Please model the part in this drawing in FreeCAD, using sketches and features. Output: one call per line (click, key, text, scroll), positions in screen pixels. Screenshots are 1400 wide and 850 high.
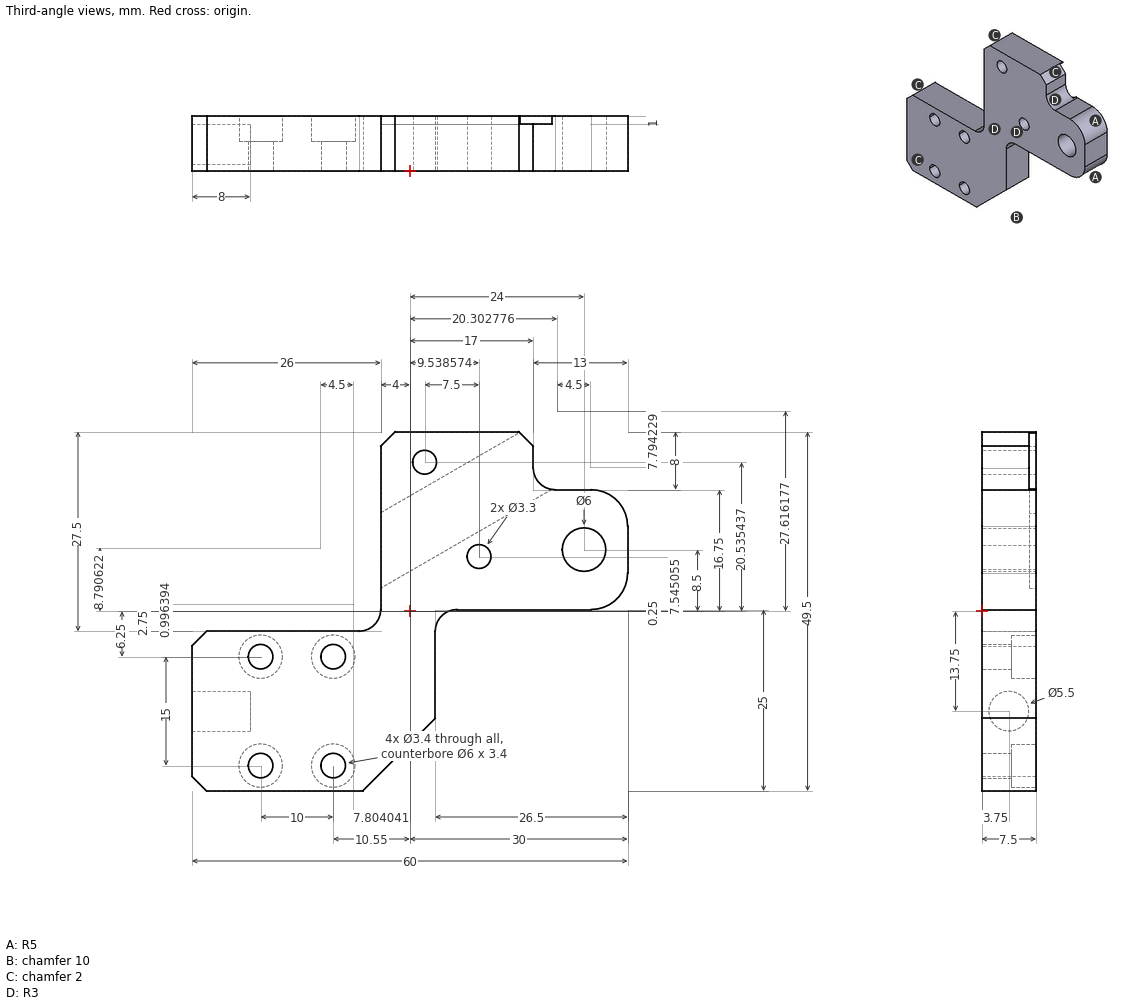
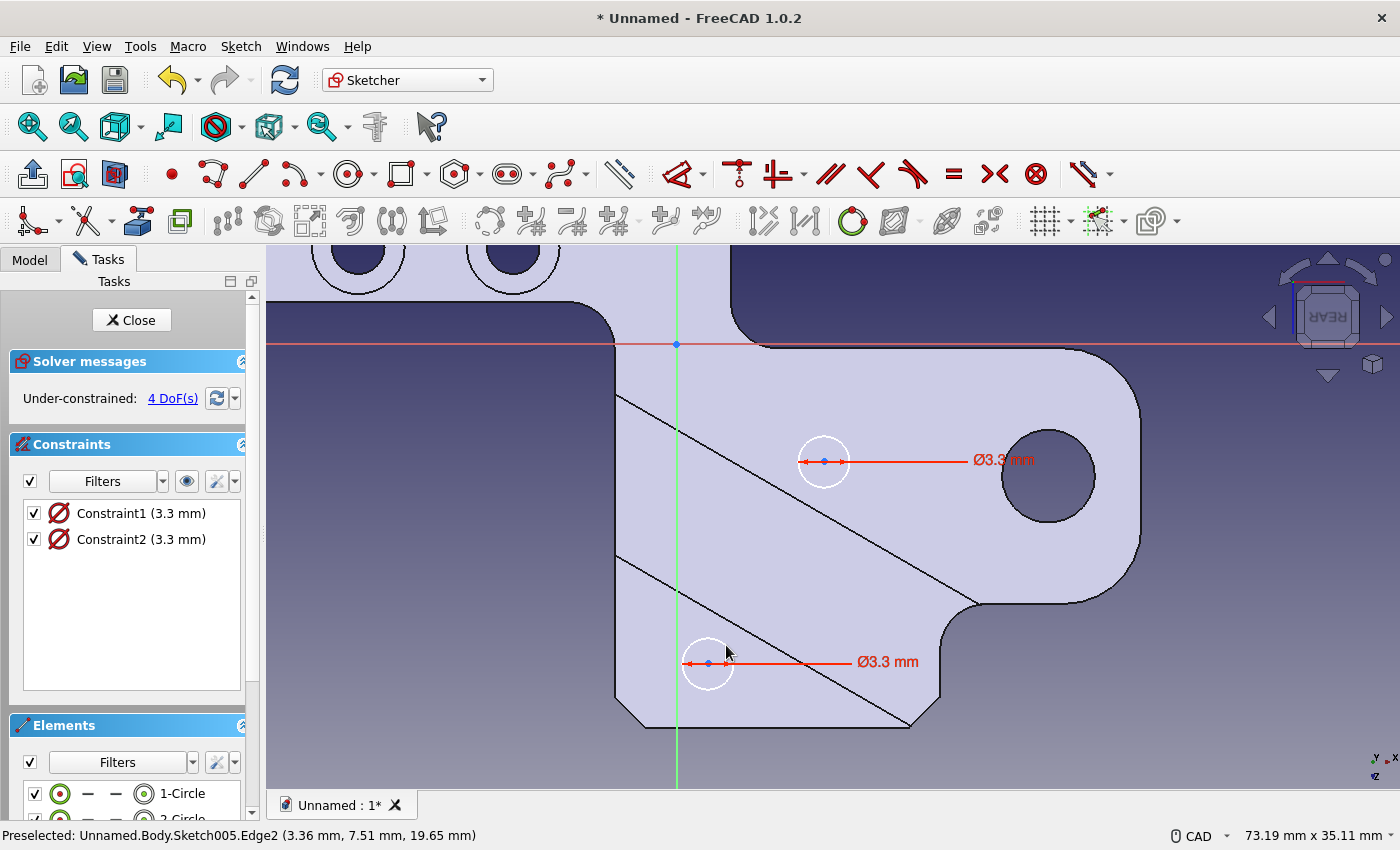
key(d)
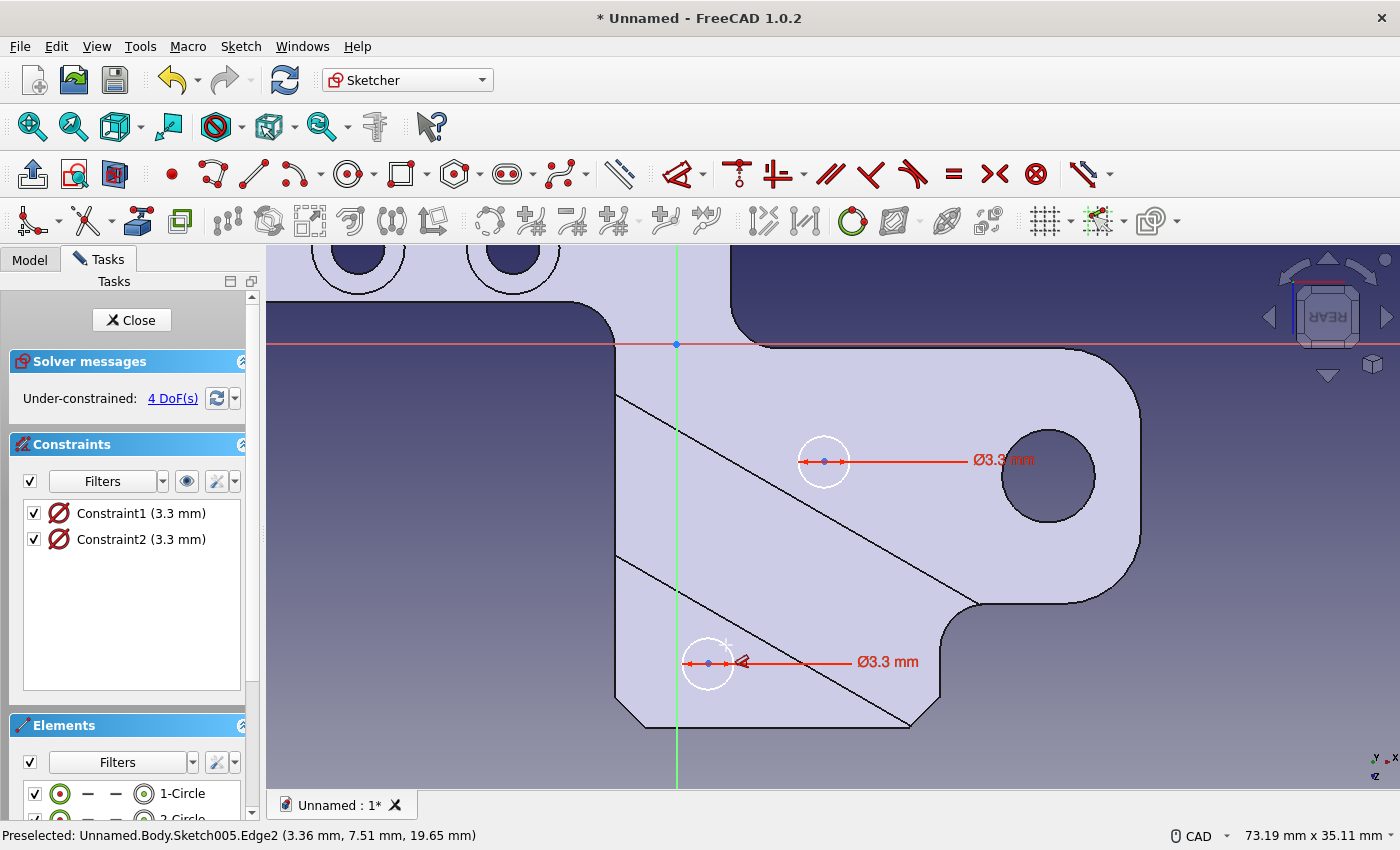
click(824, 462)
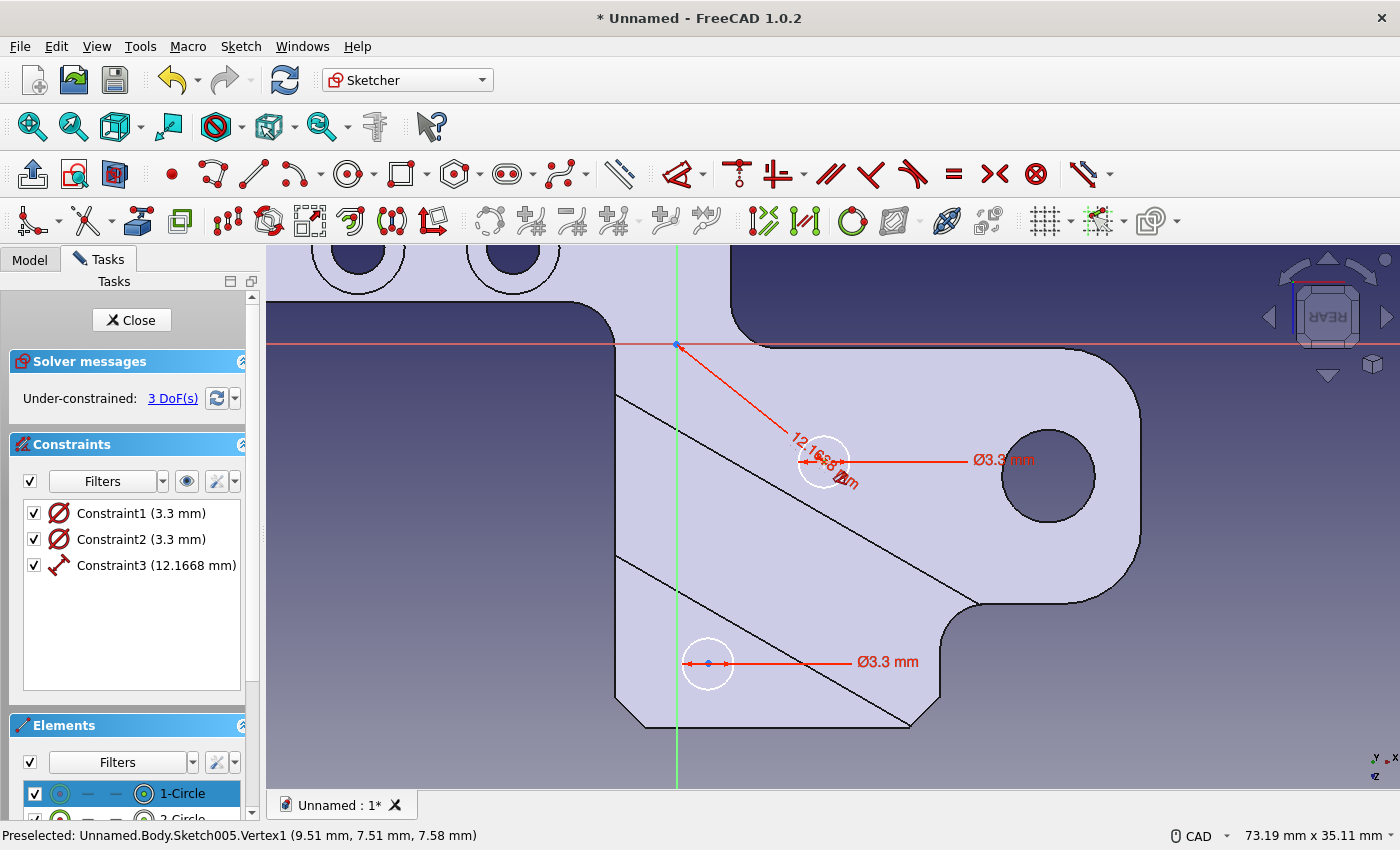
click(708, 664)
click(766, 698)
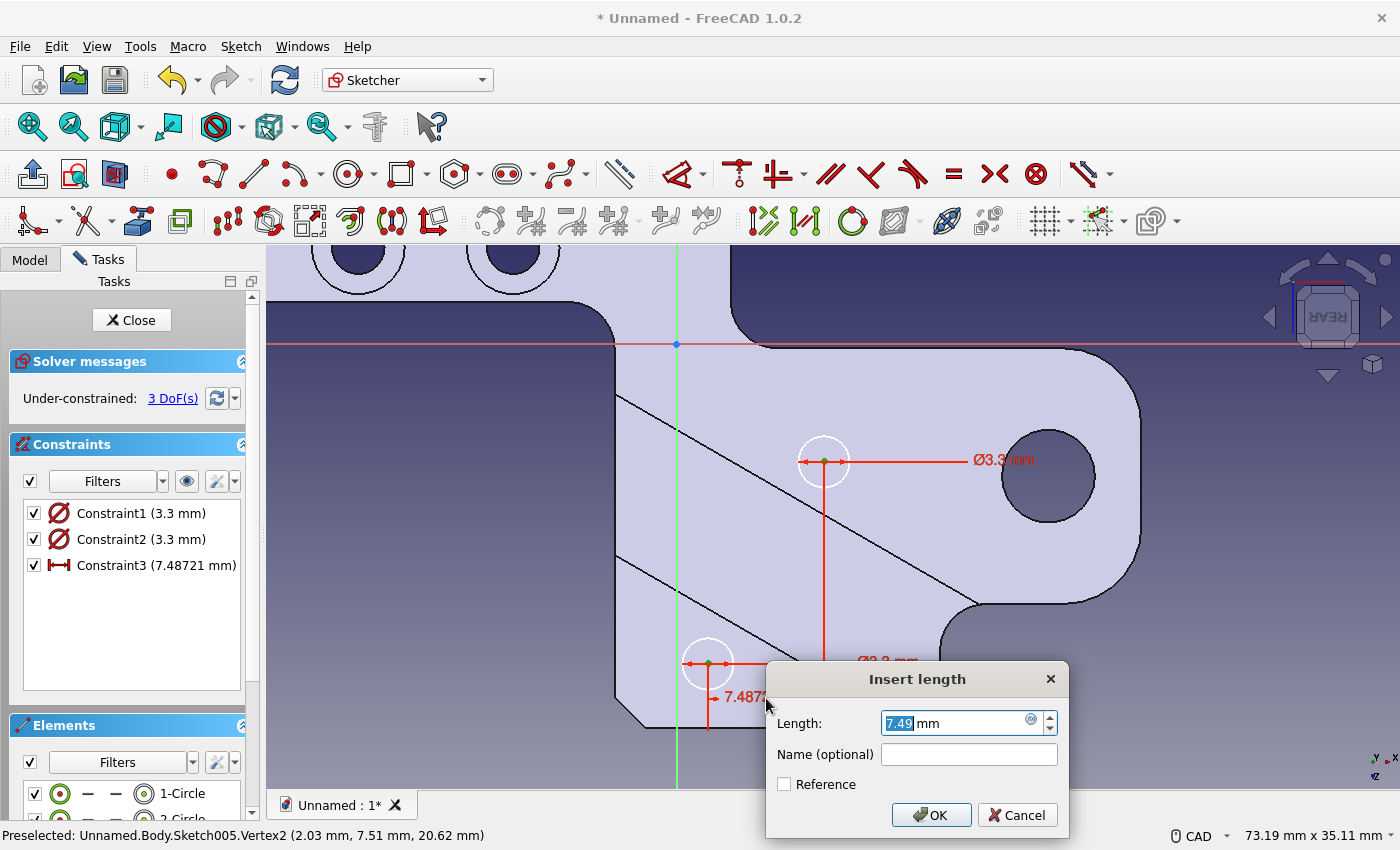
text(7.5)
key(Return)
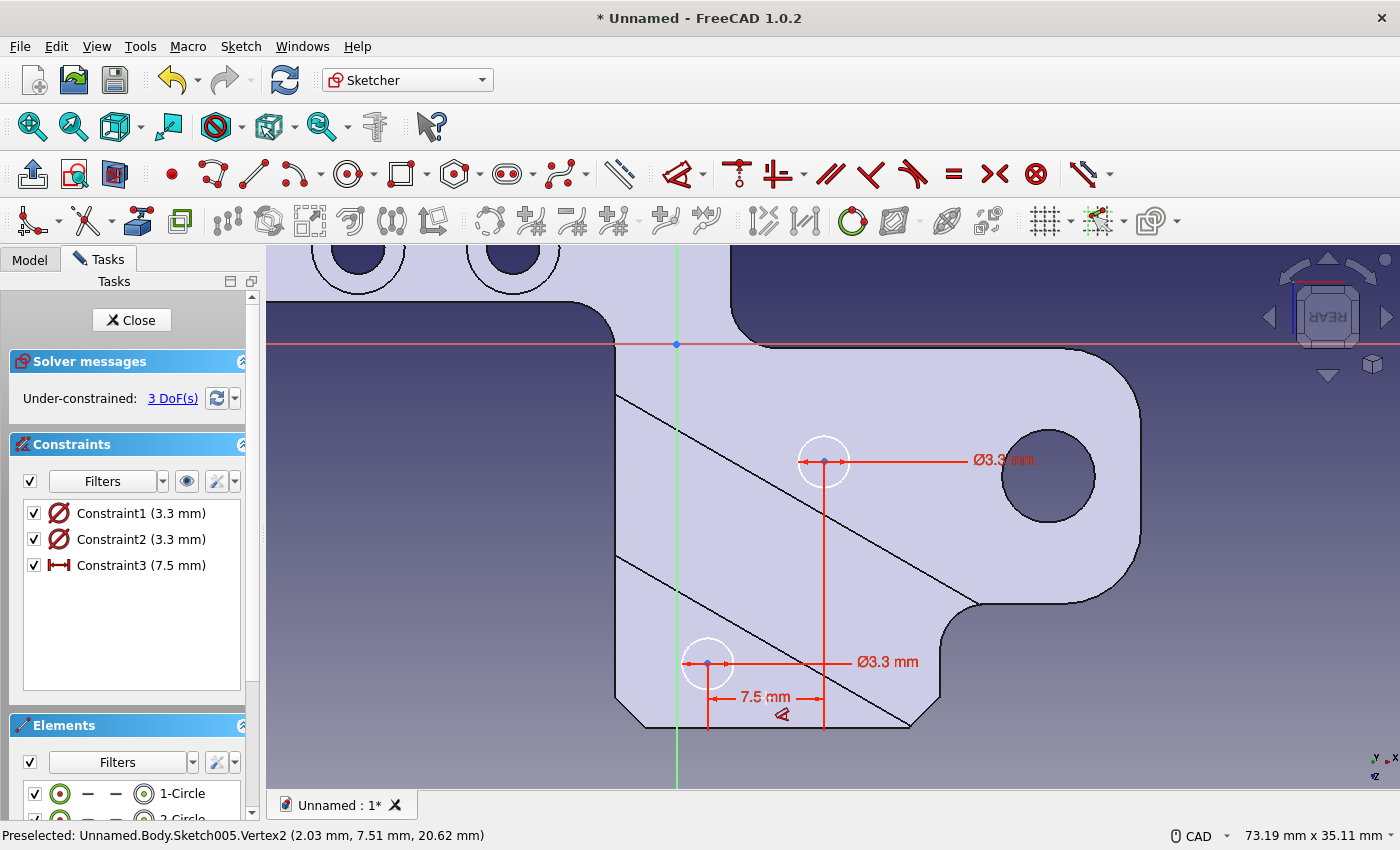
click(824, 462)
click(750, 310)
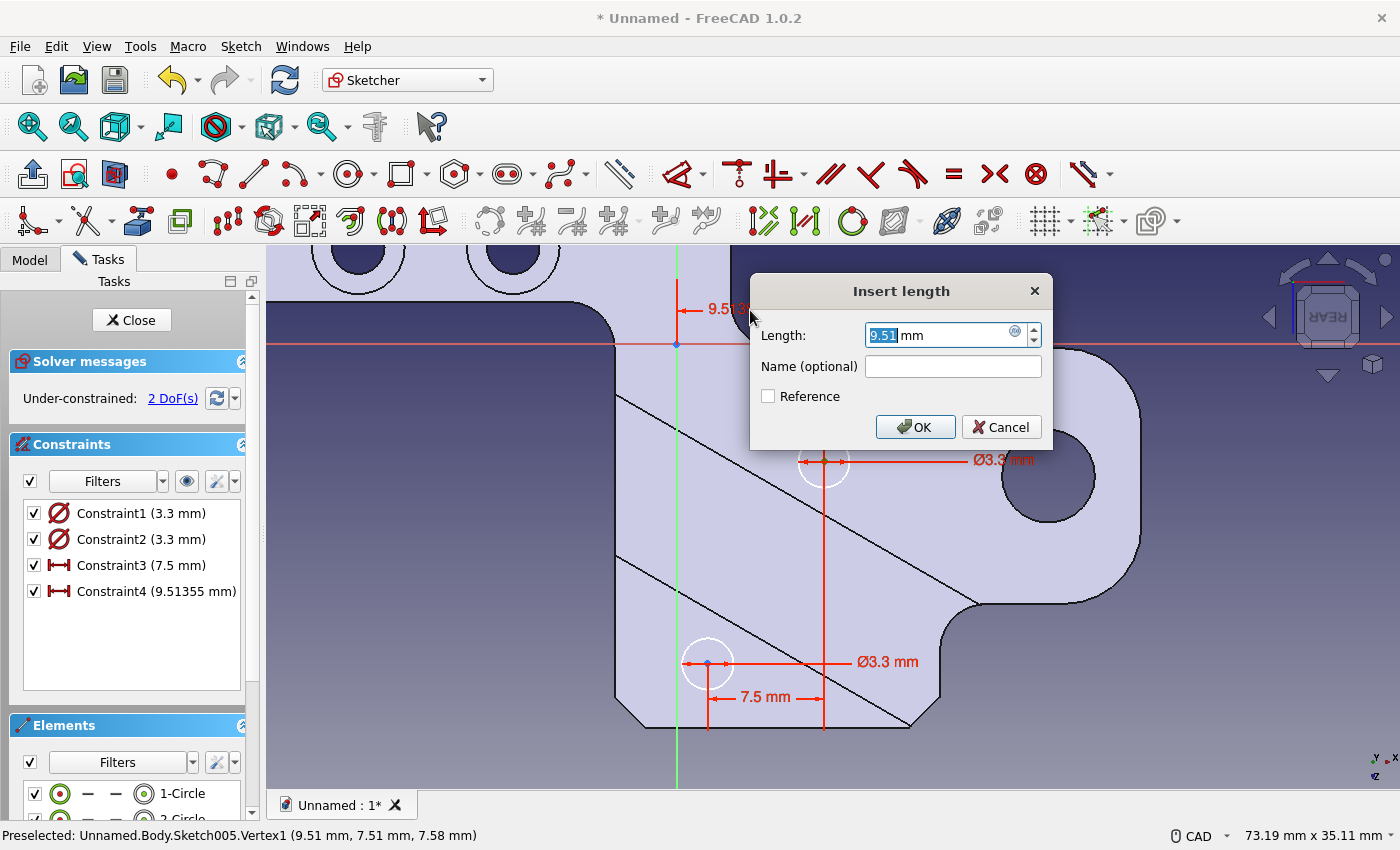
text(9.538574)
key(Return)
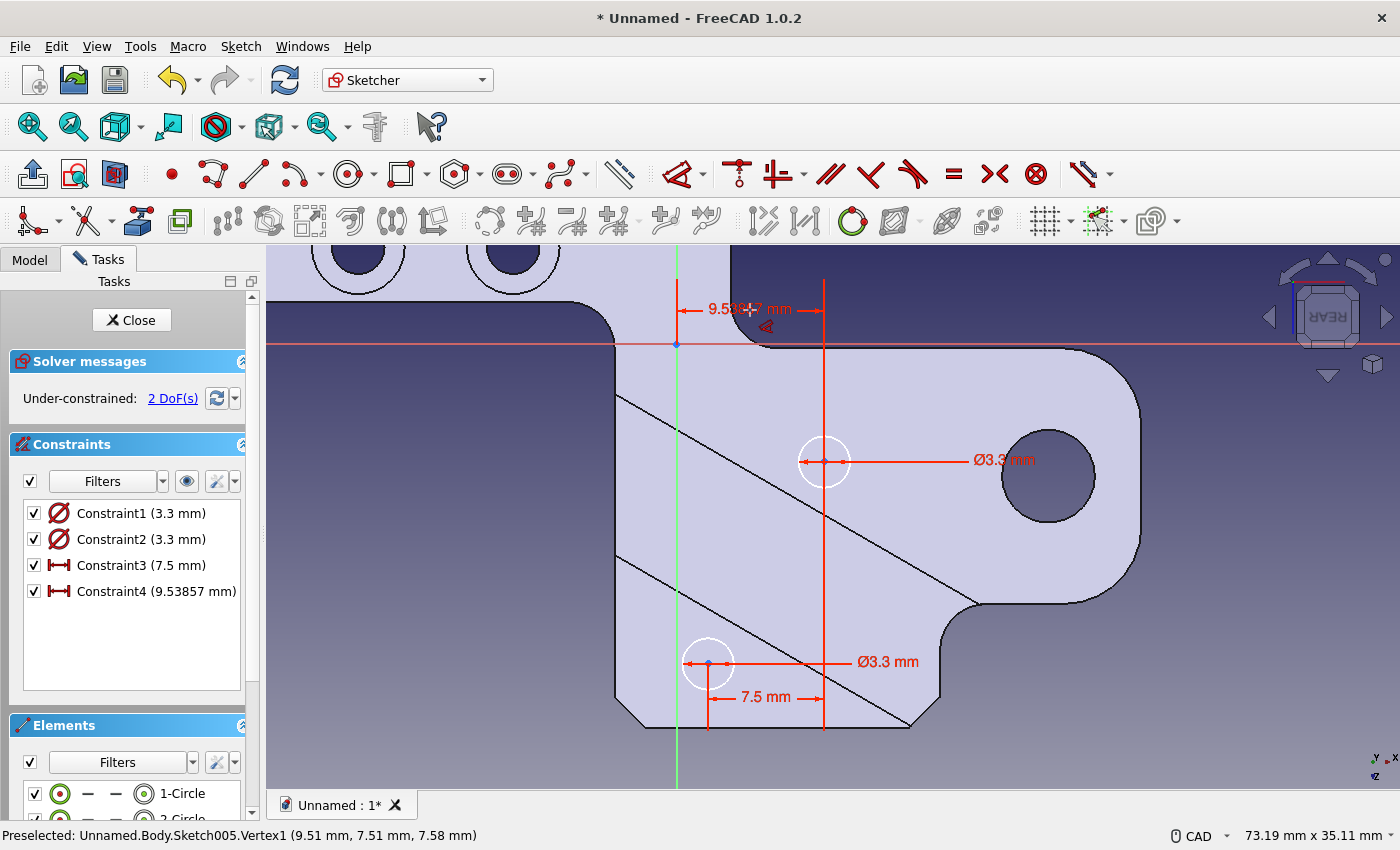
click(824, 462)
click(643, 403)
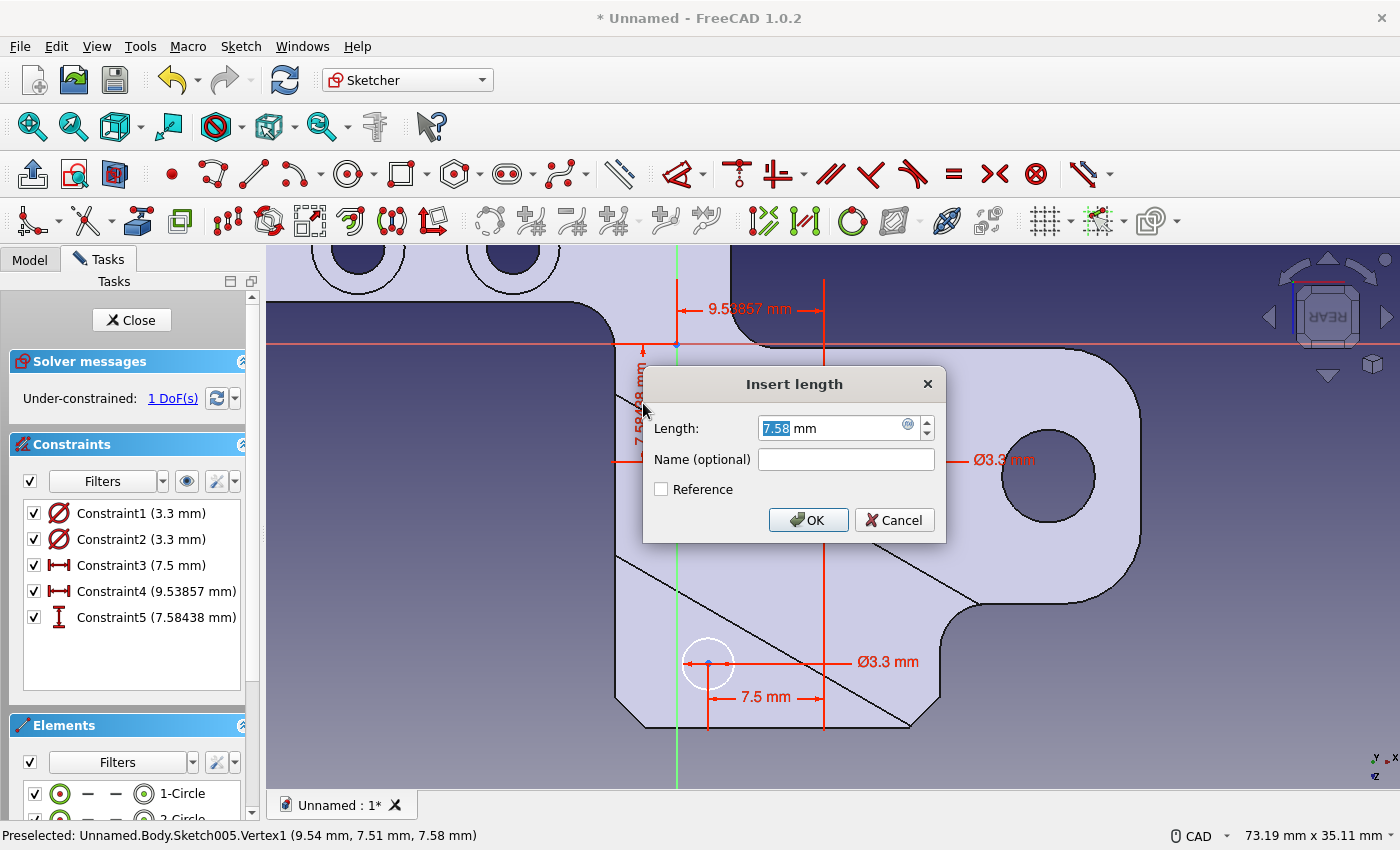
text(7.545055)
key(Return)